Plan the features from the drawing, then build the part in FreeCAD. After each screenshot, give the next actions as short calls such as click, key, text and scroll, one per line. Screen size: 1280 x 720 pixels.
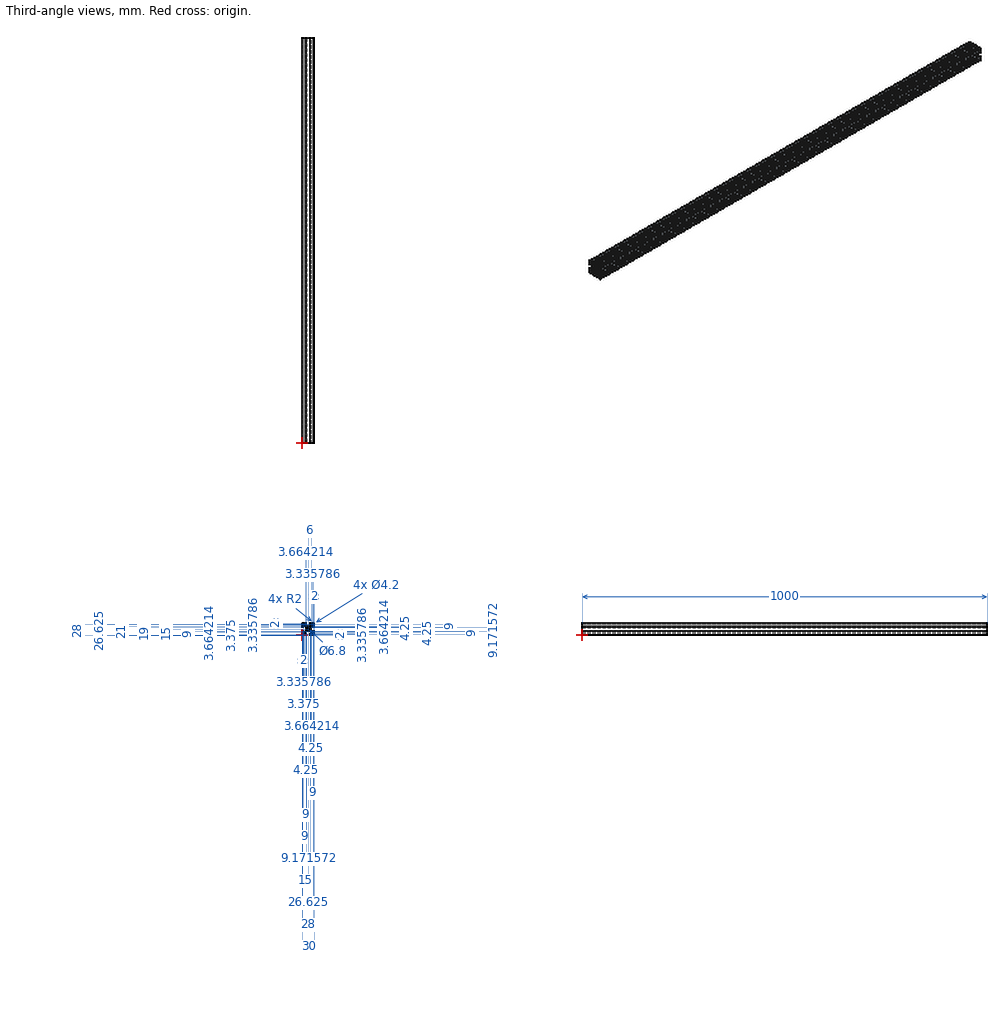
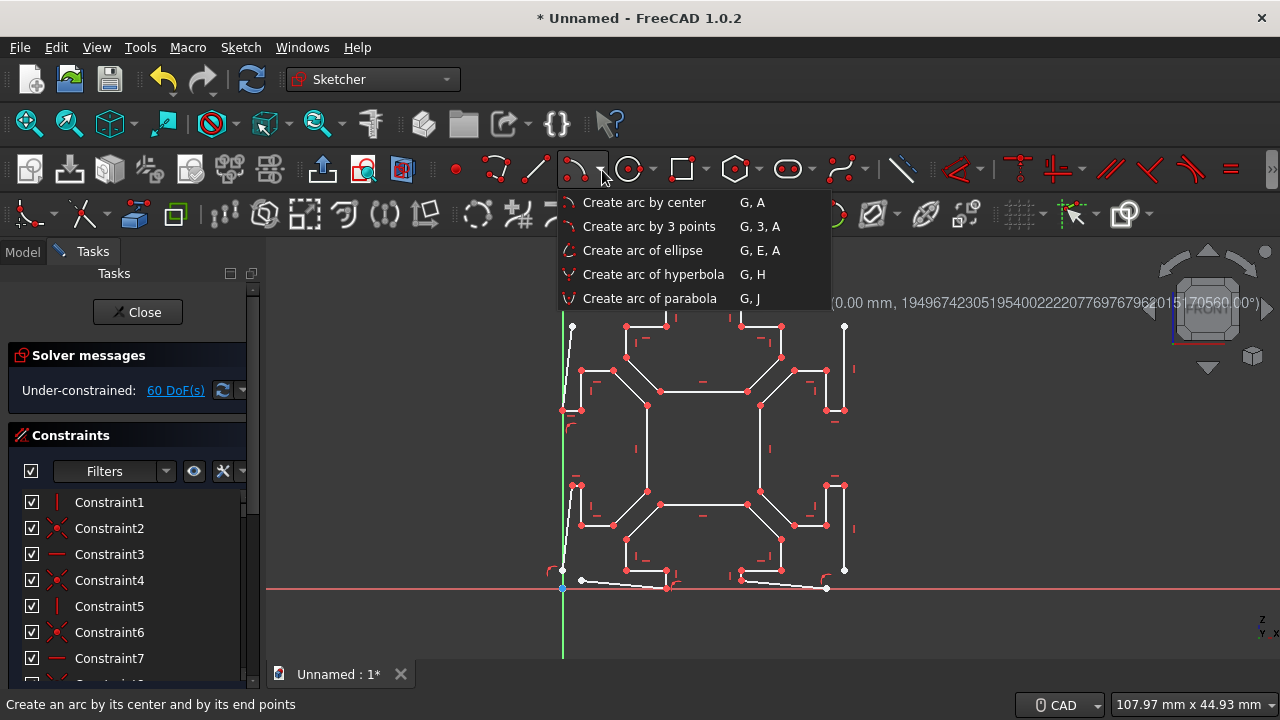
click(694, 226)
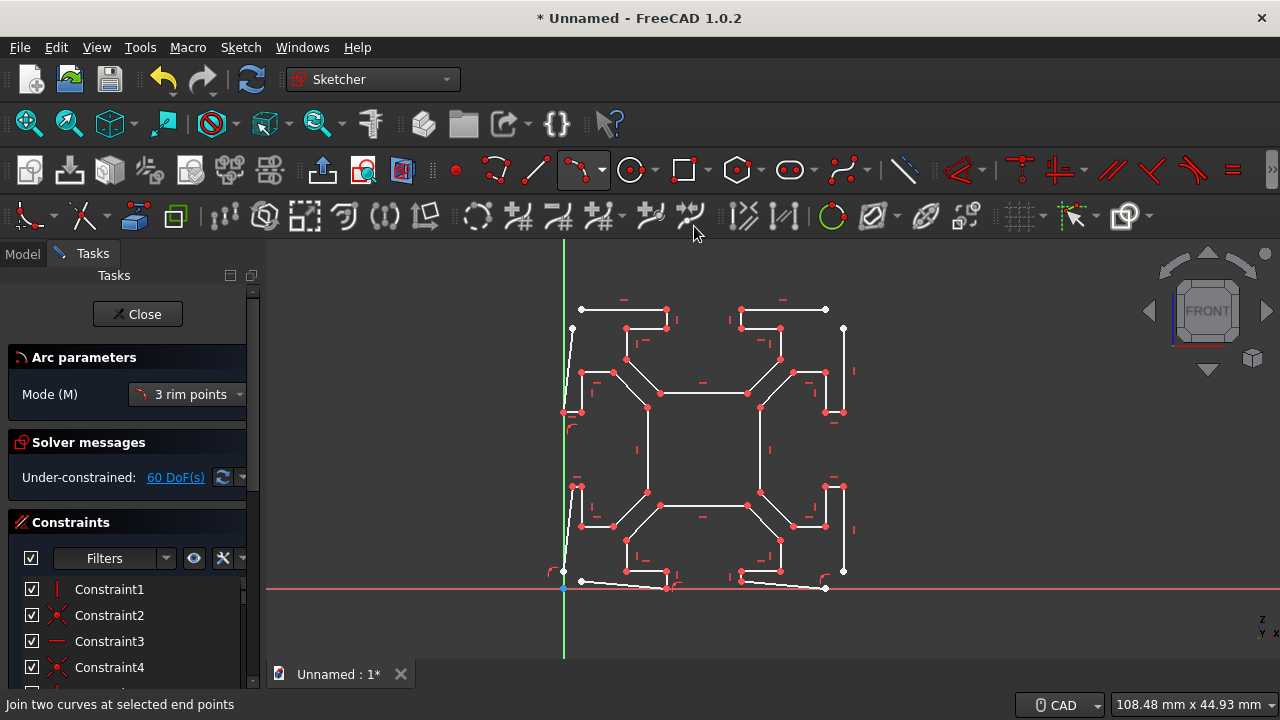
click(844, 571)
click(826, 589)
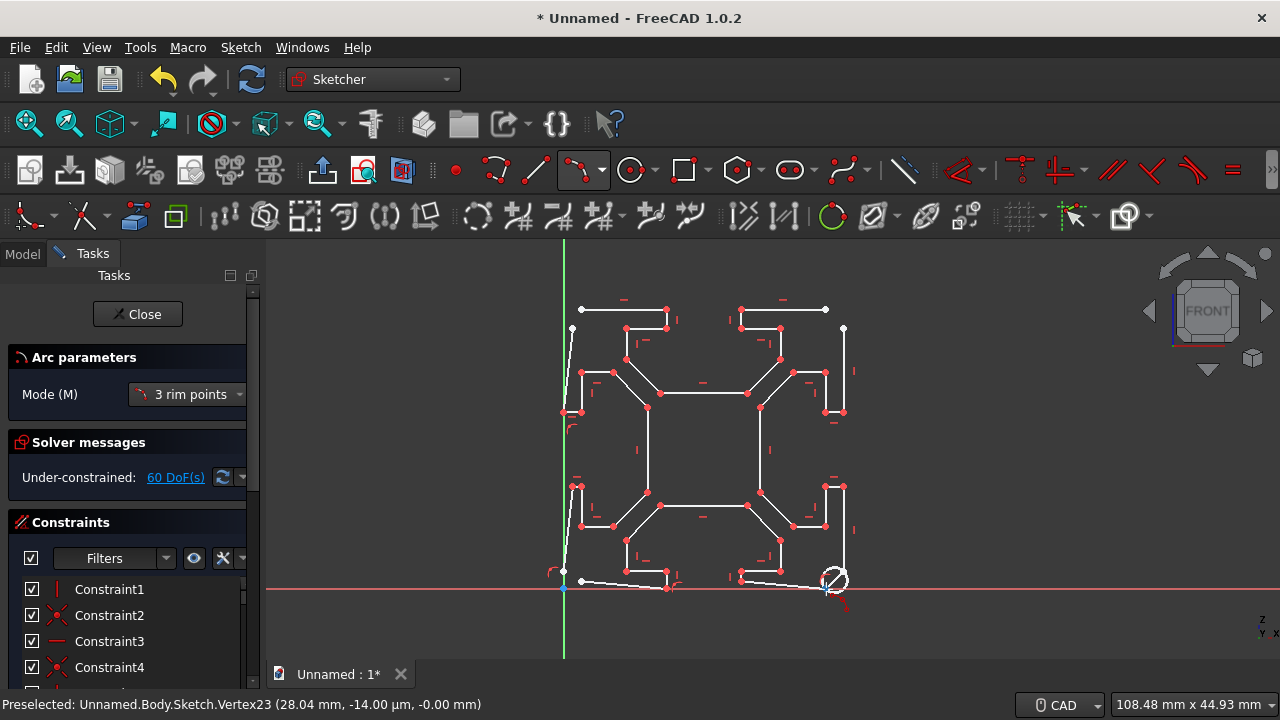
scroll(839, 584, up, 6)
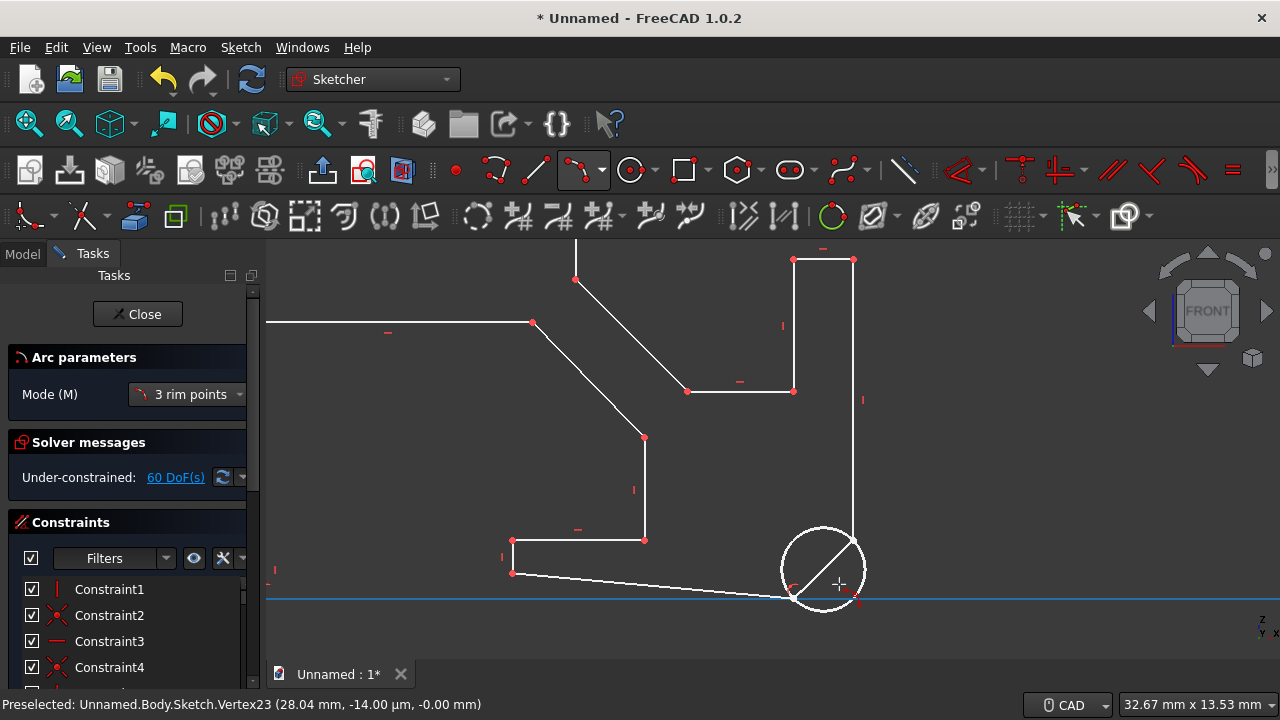
click(836, 580)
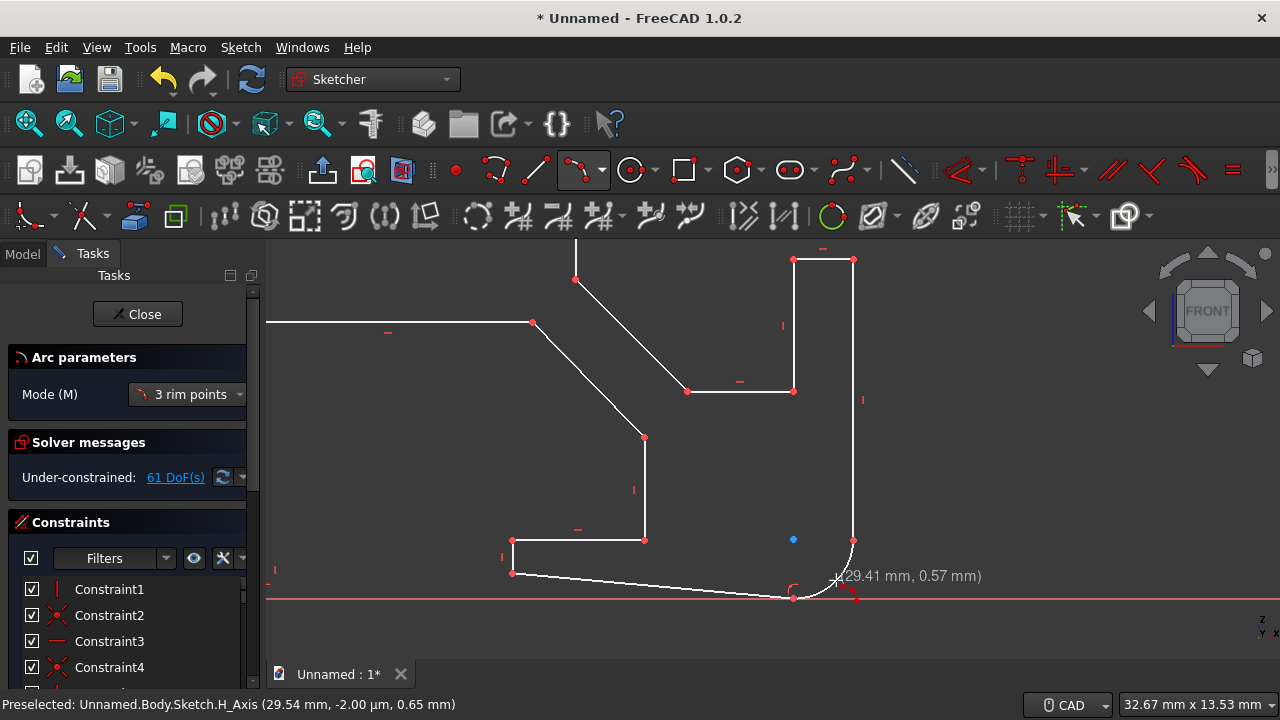
scroll(841, 585, down, 6)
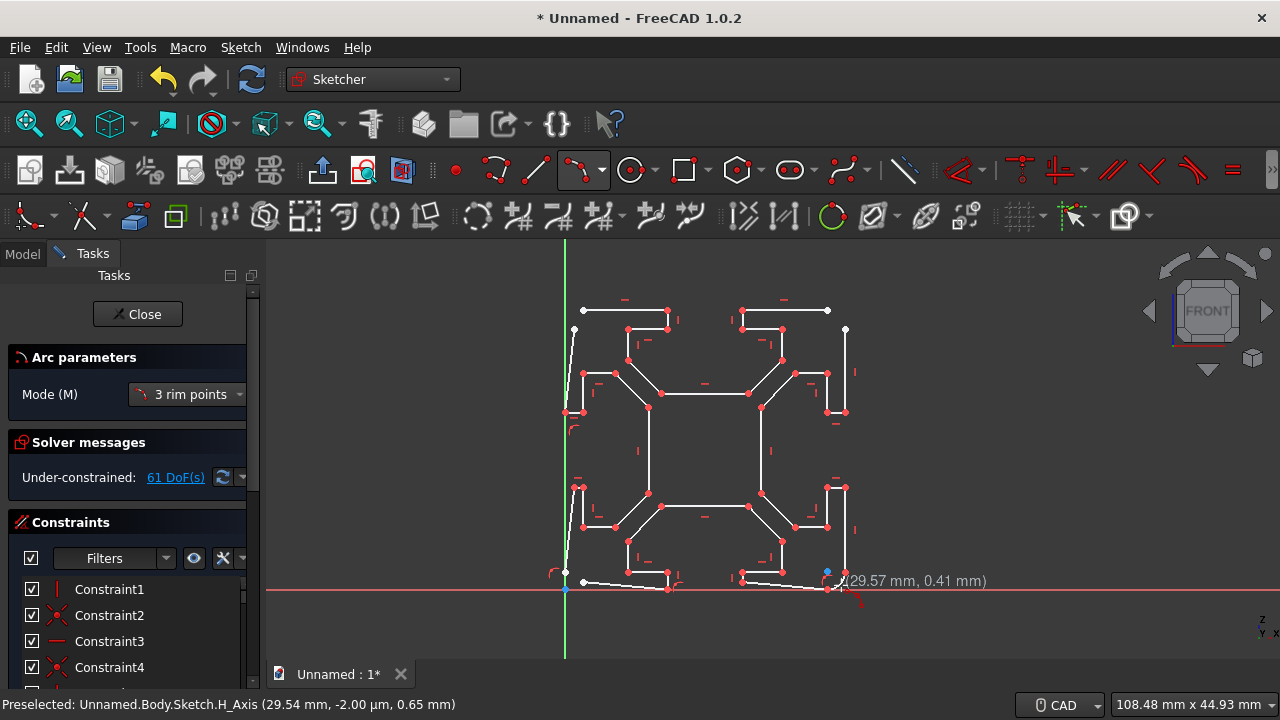
click(583, 582)
click(565, 572)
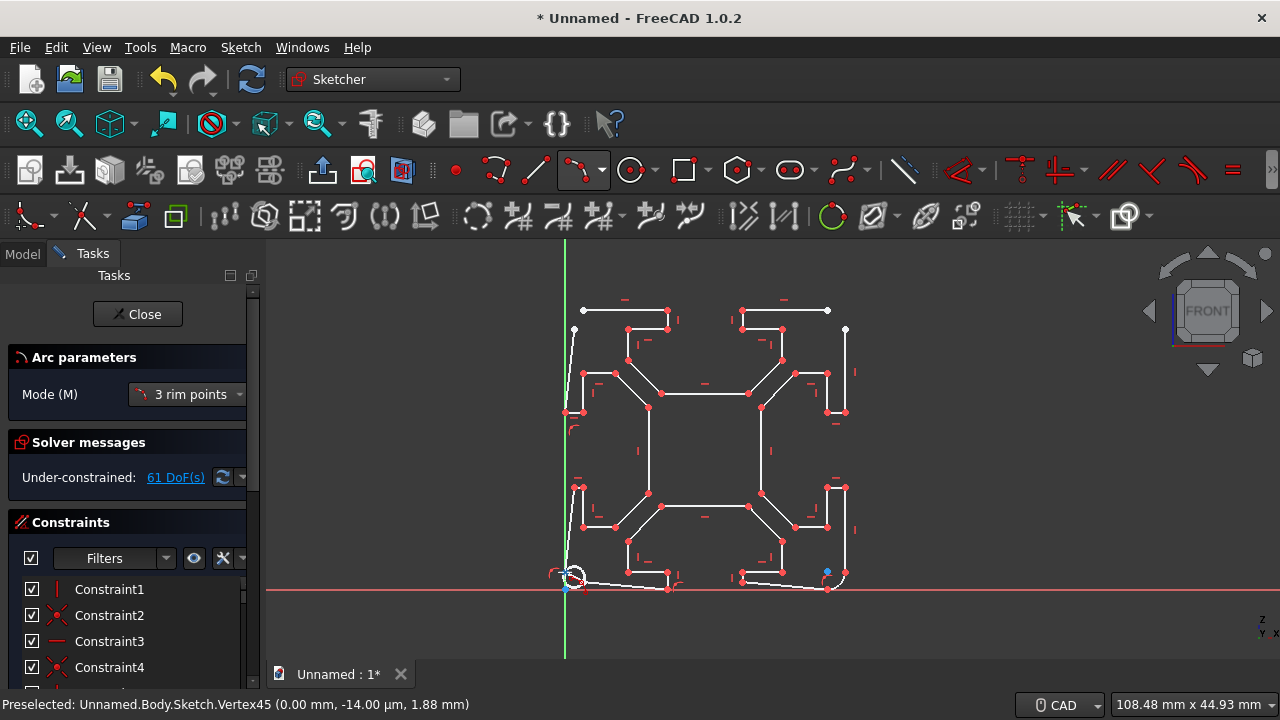
scroll(570, 584, up, 6)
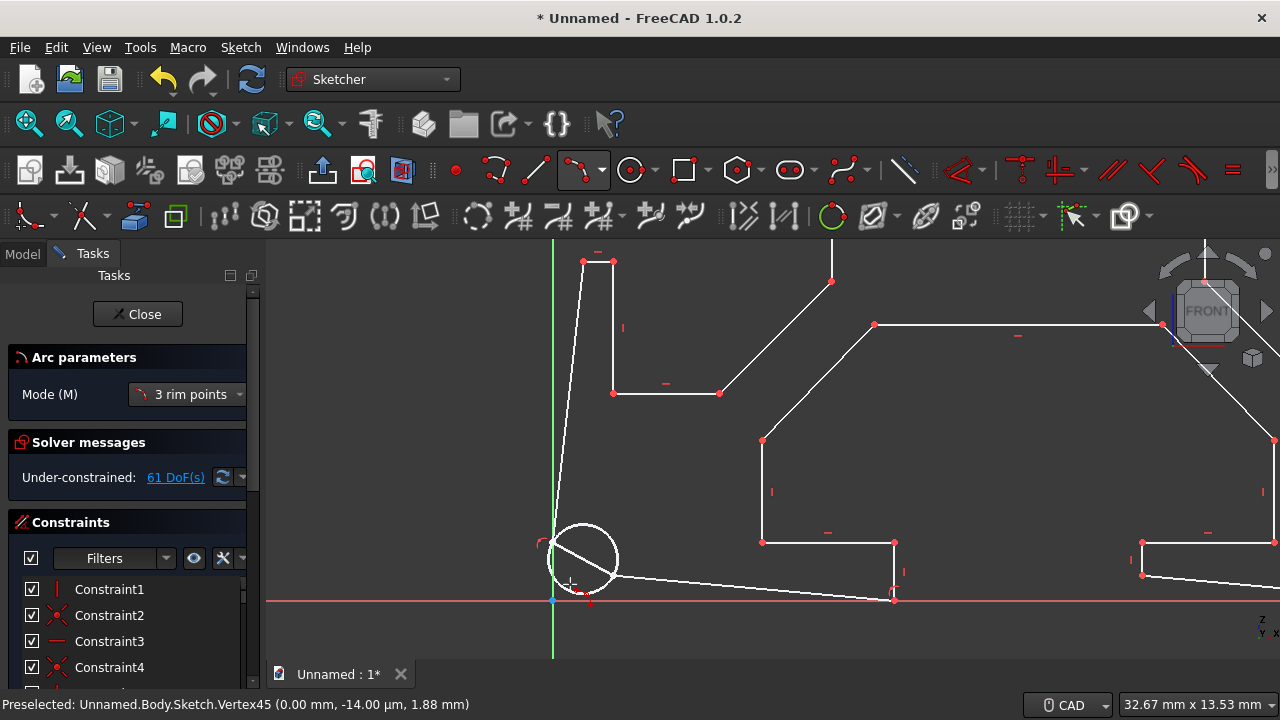
click(571, 583)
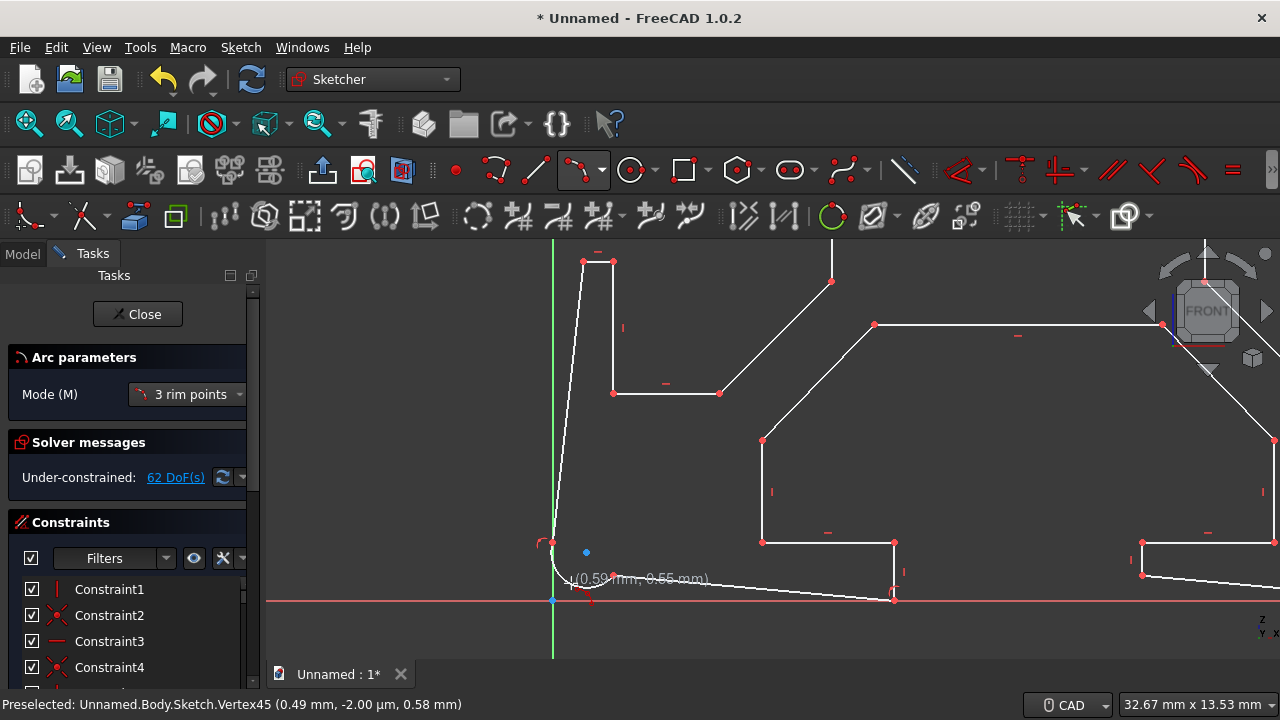
scroll(569, 584, down, 6)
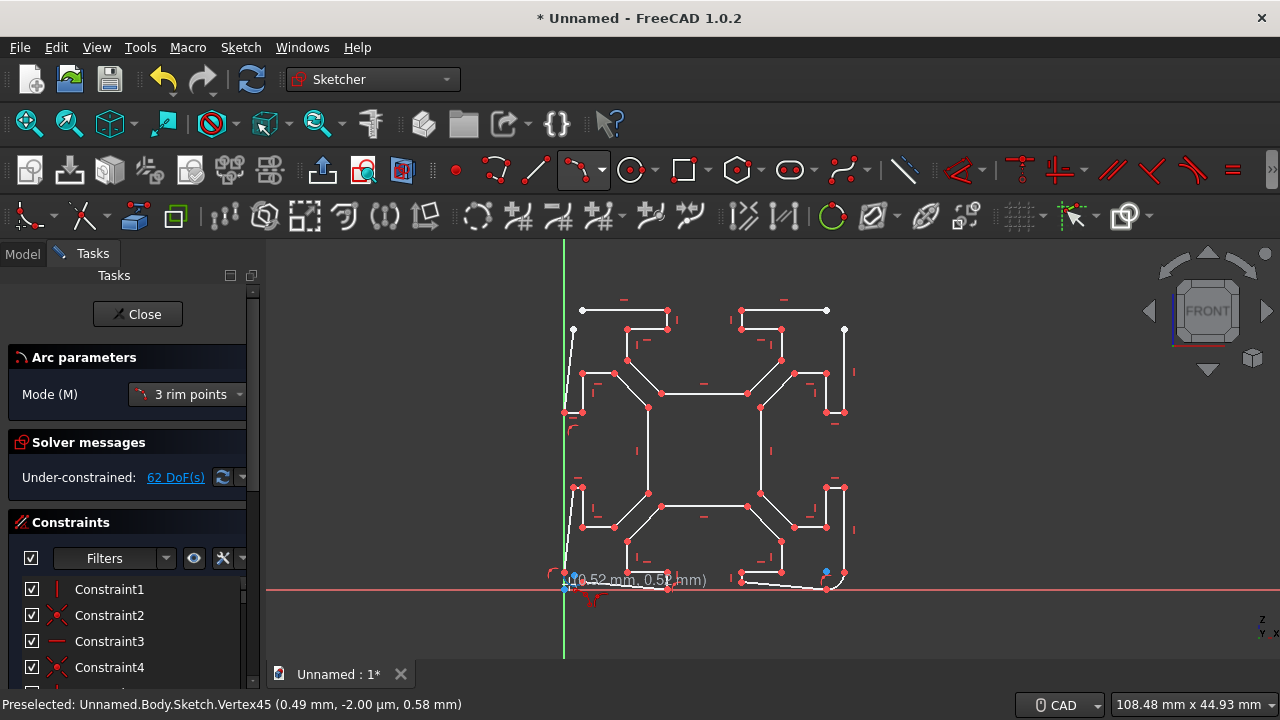
click(574, 329)
click(583, 310)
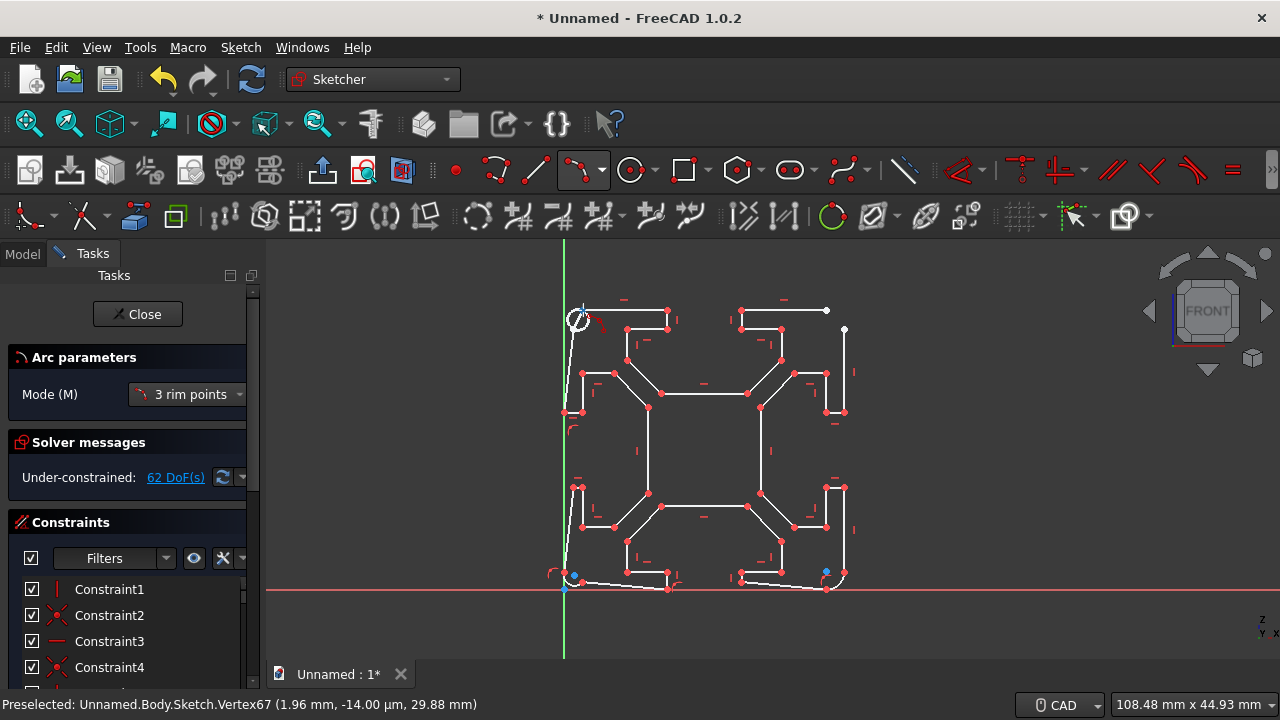
scroll(570, 315, up, 6)